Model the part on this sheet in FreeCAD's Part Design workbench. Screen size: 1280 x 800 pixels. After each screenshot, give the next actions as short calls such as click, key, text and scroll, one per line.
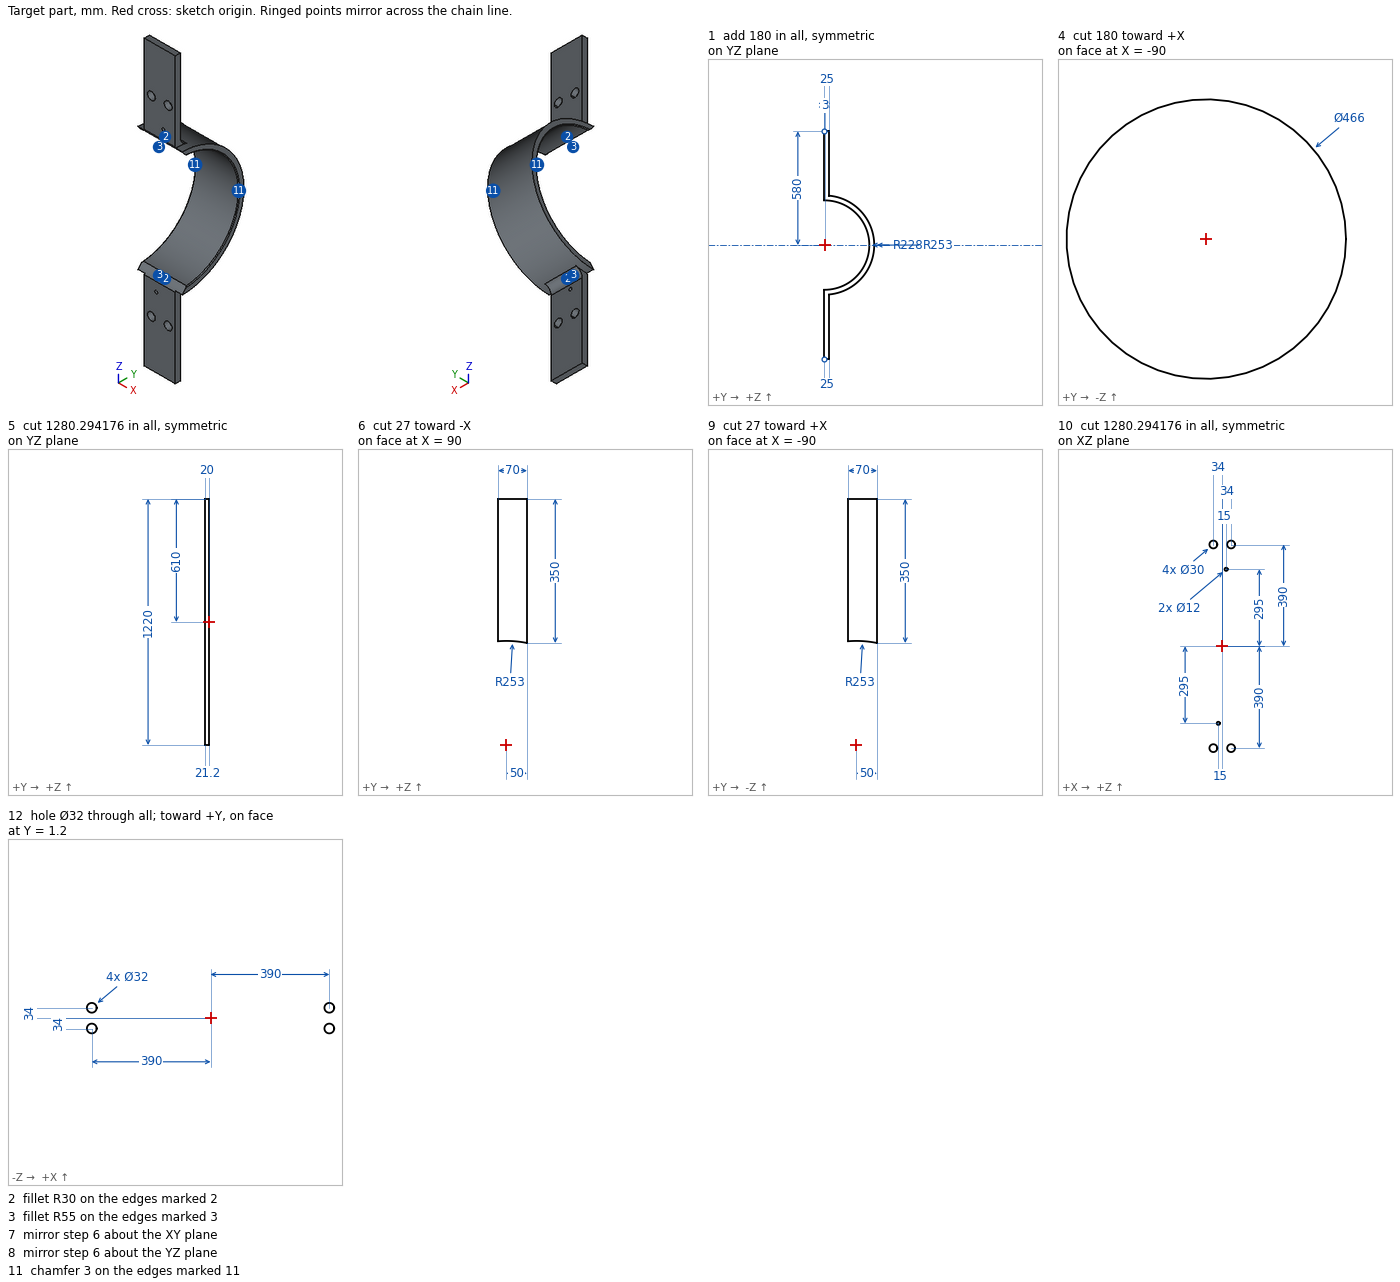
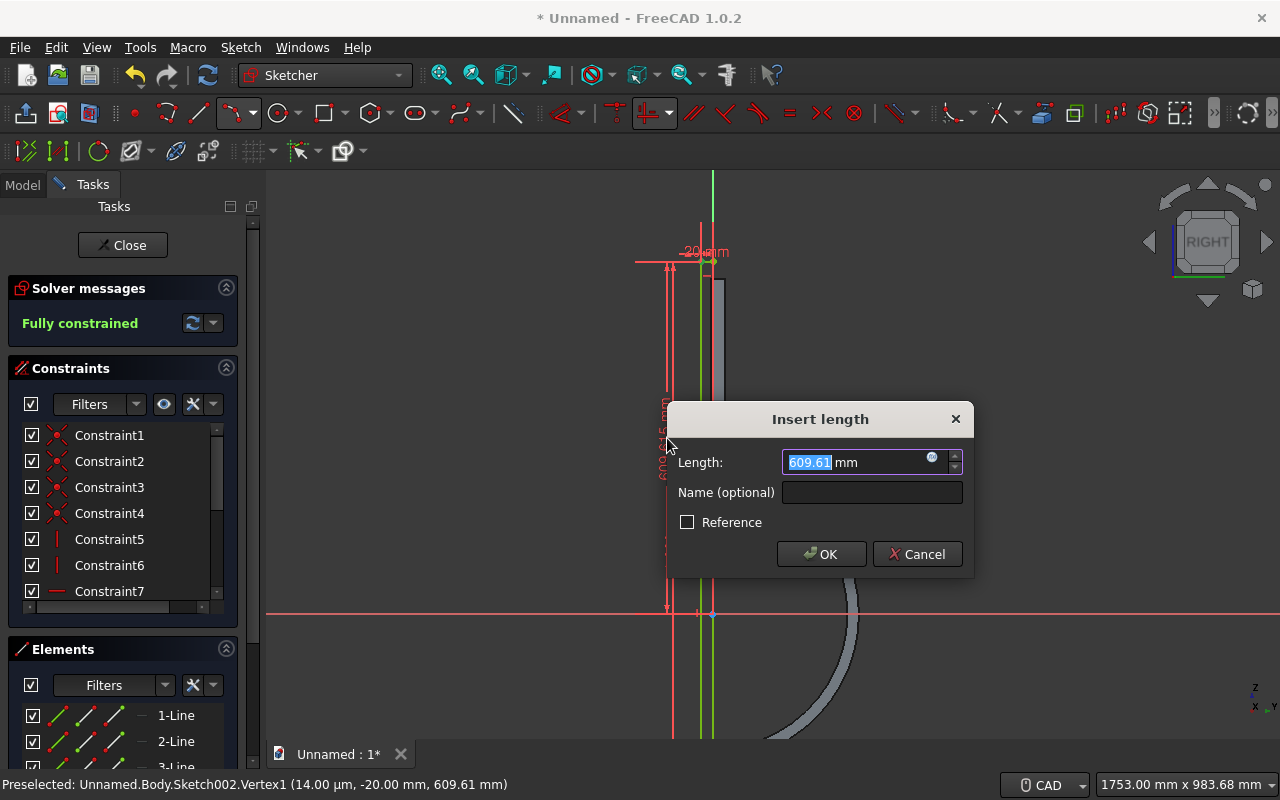
text(610)
key(Return)
key(Escape)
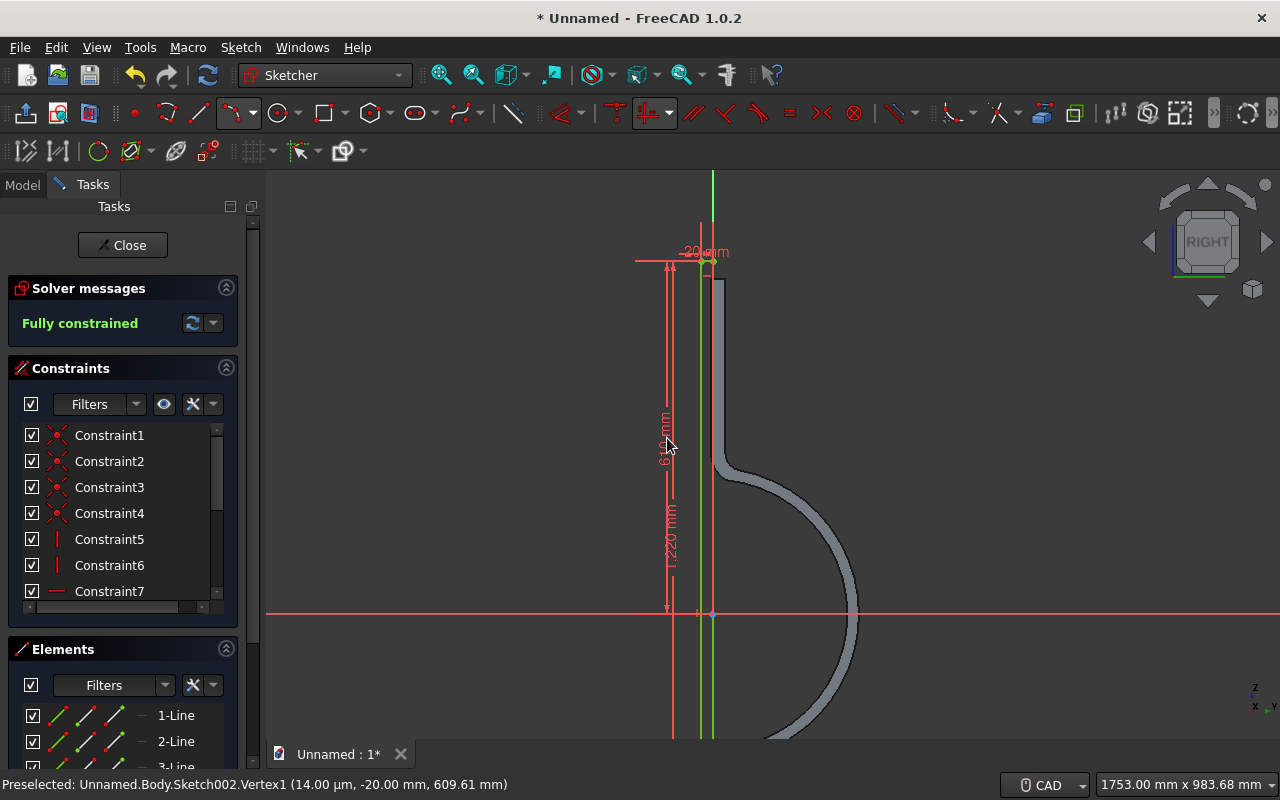
click(123, 245)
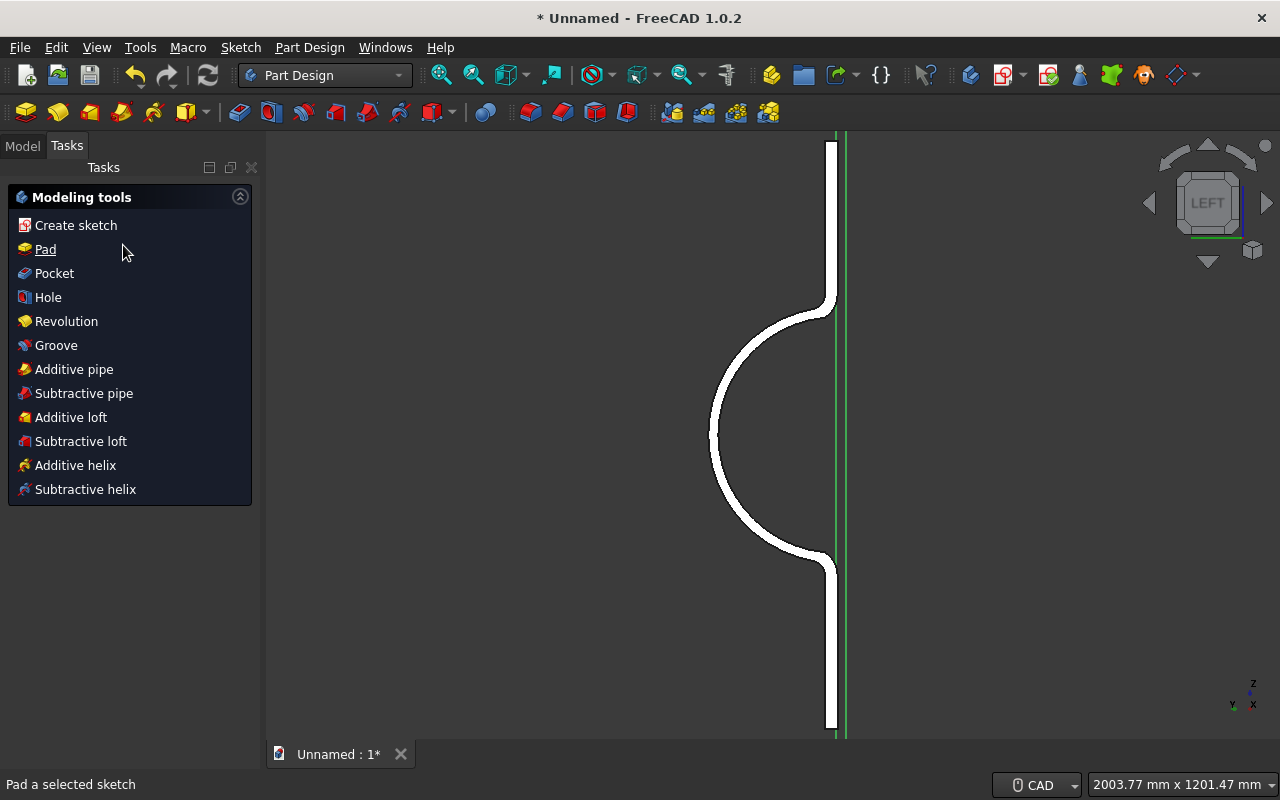
click(240, 112)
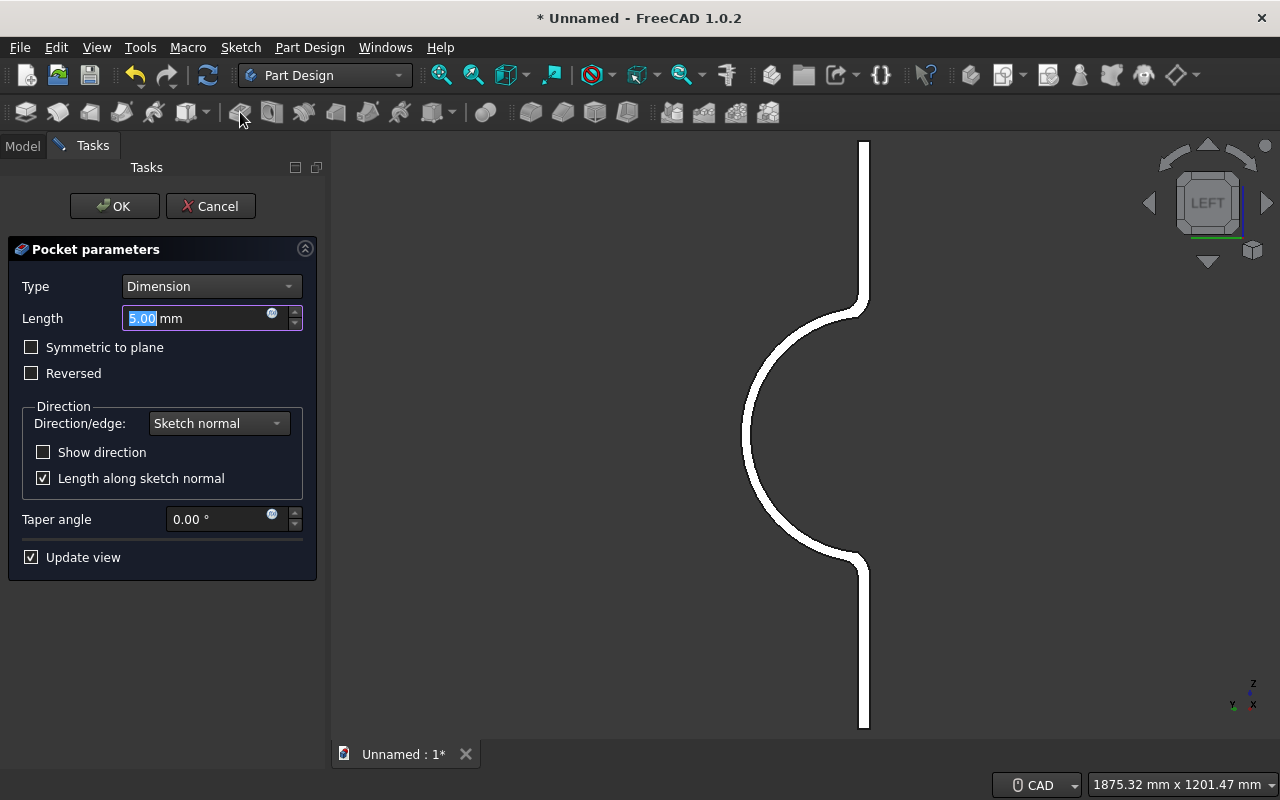
text(1280.294176)
key(Tab)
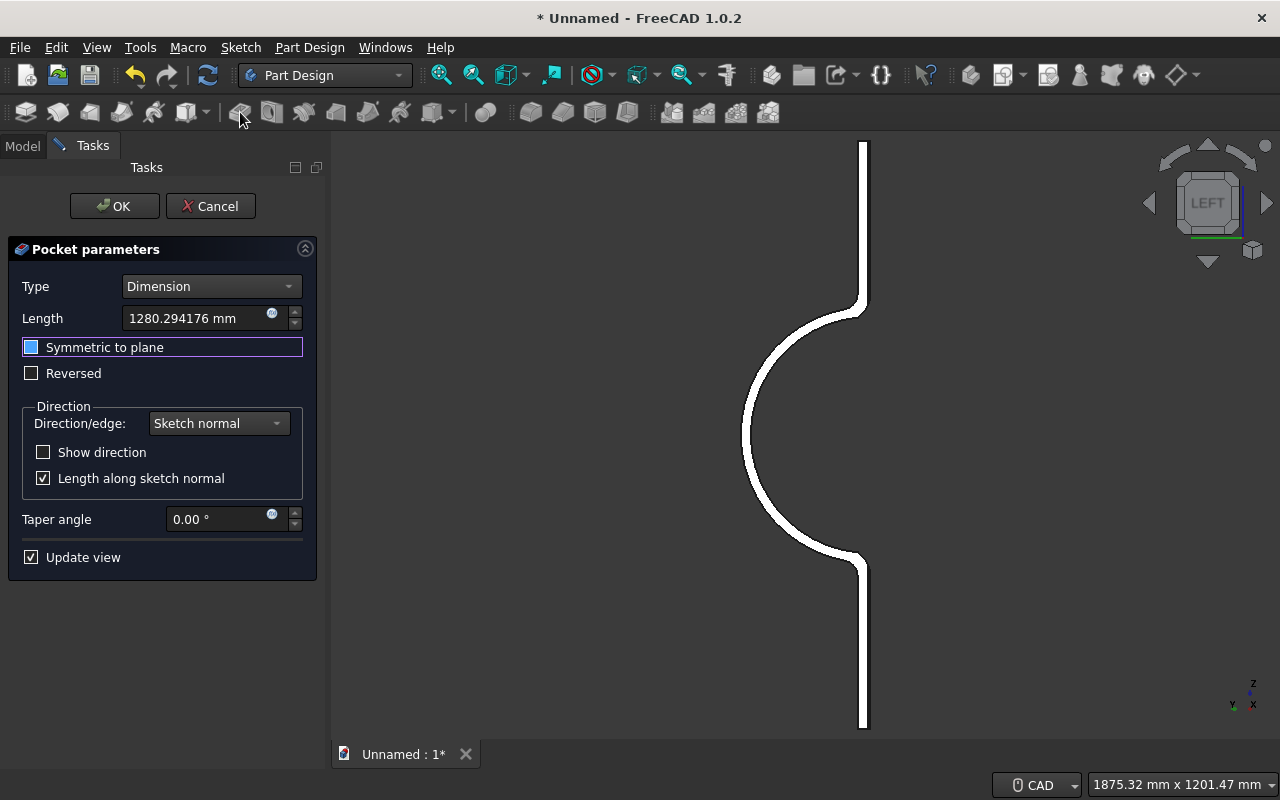
click(30, 347)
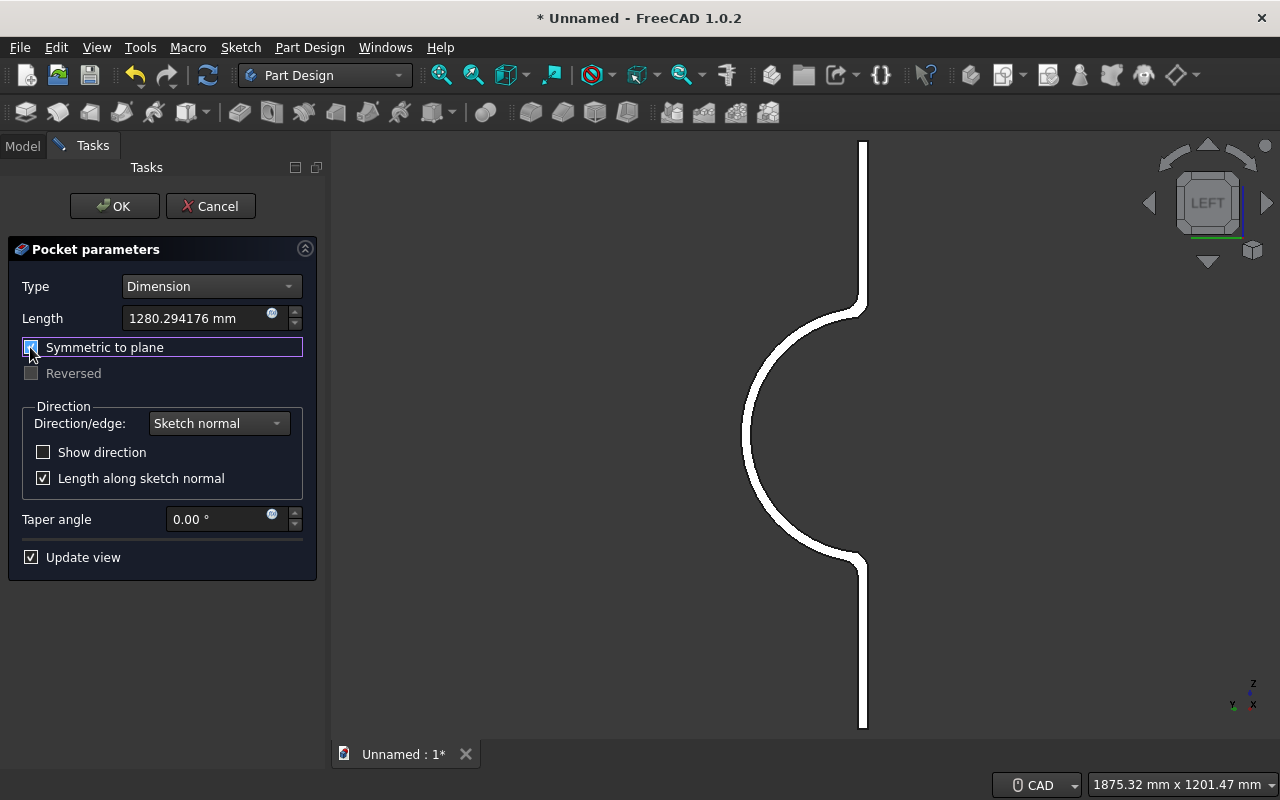
click(115, 206)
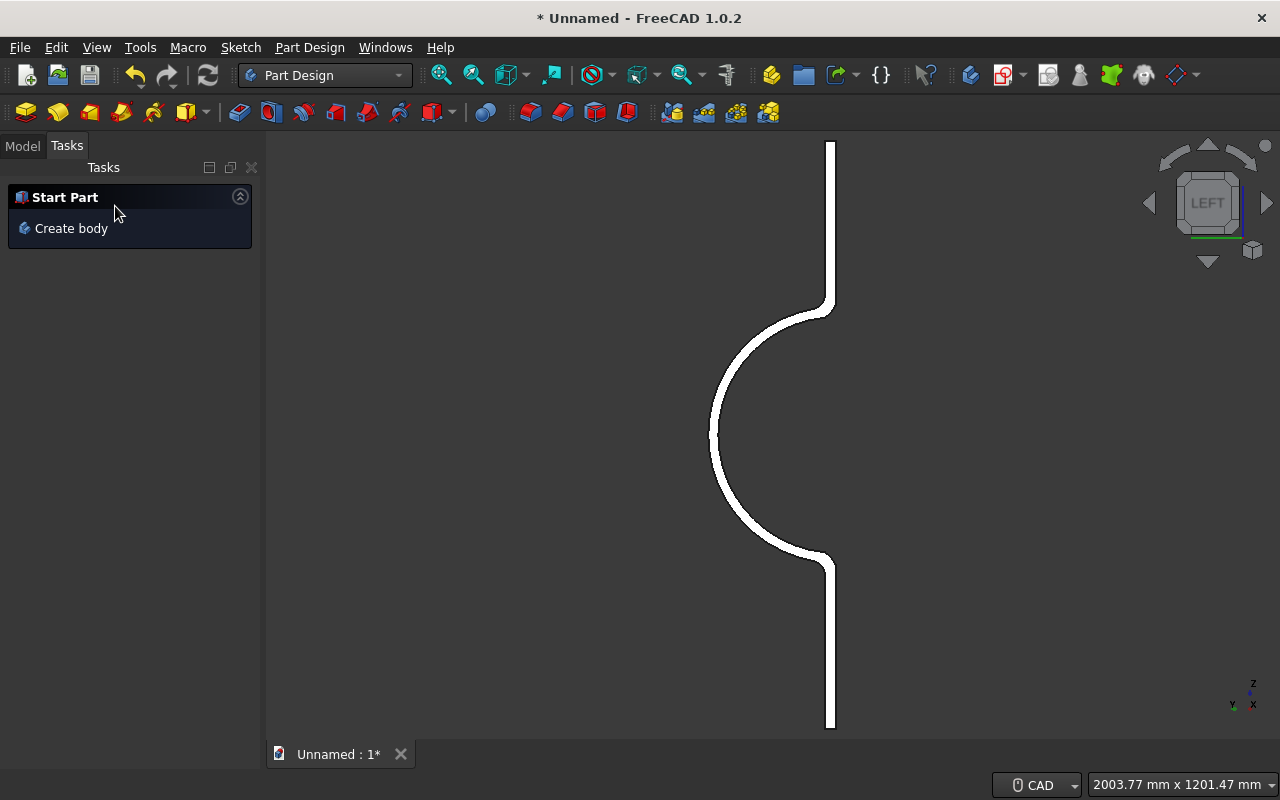
key(0)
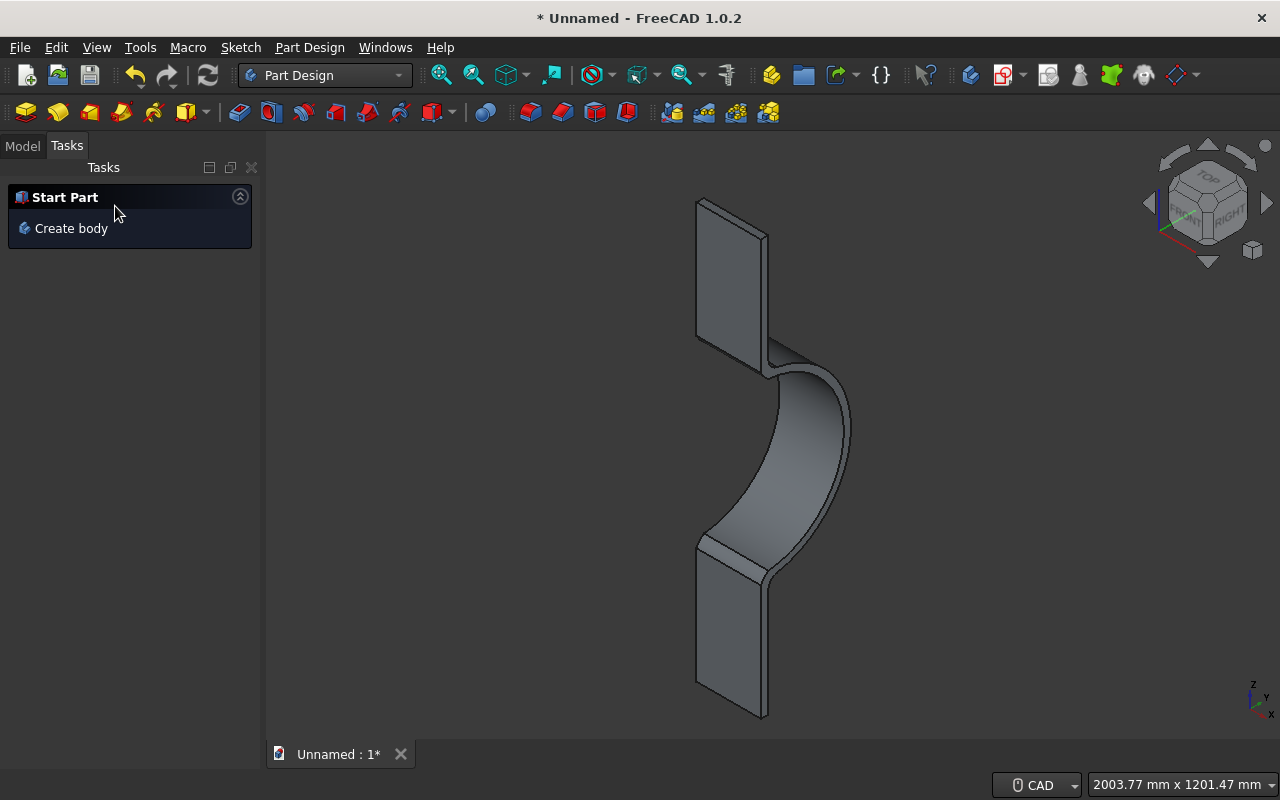
scroll(767, 338, up, 11)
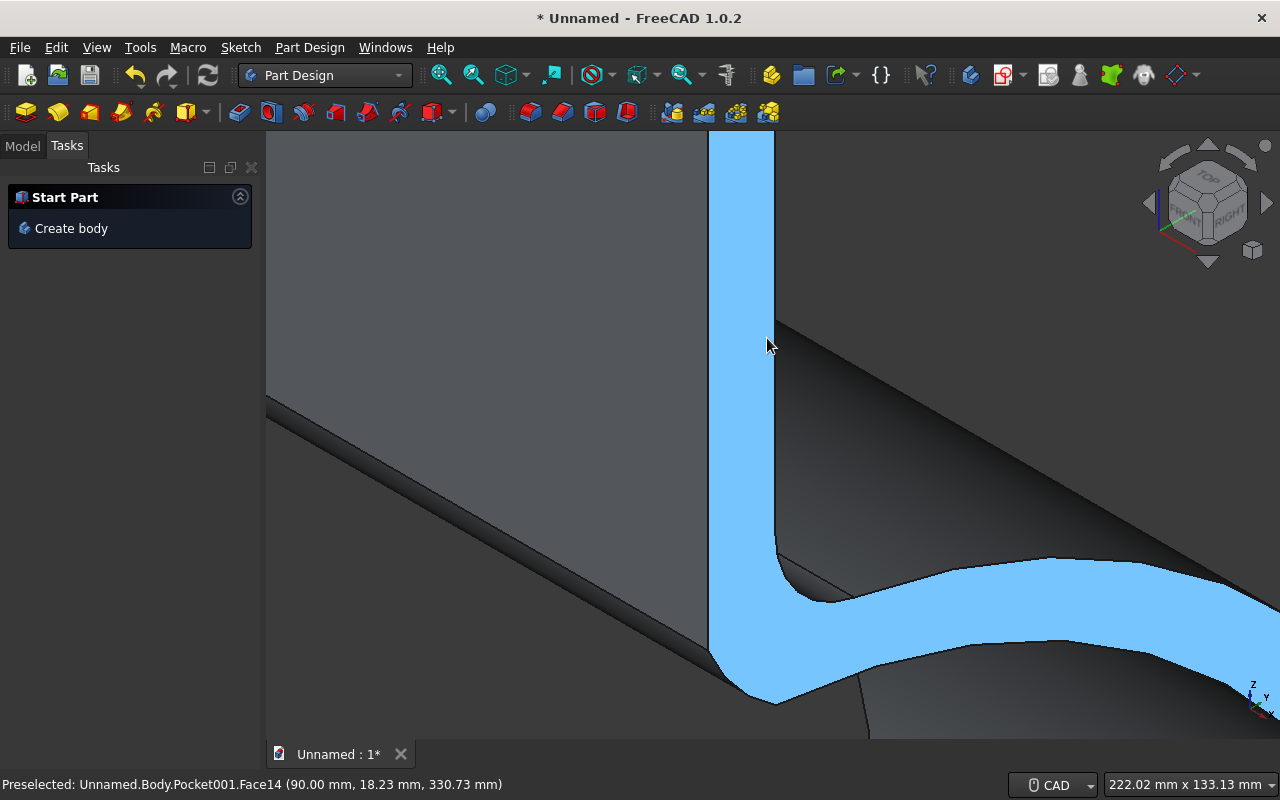
click(766, 339)